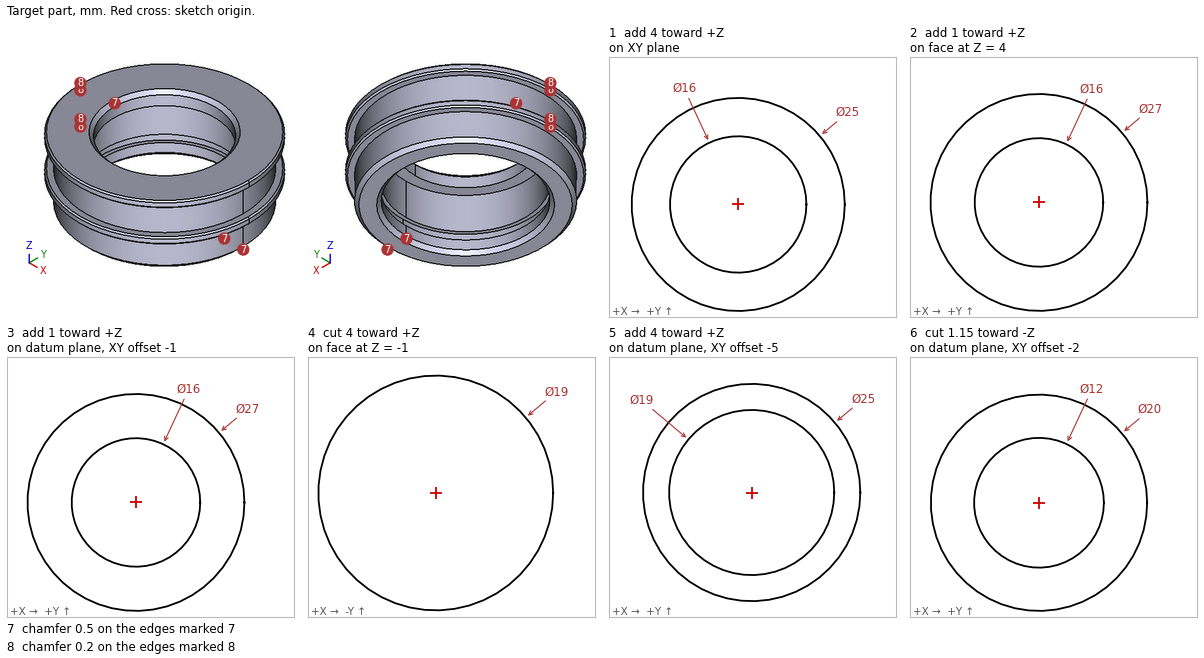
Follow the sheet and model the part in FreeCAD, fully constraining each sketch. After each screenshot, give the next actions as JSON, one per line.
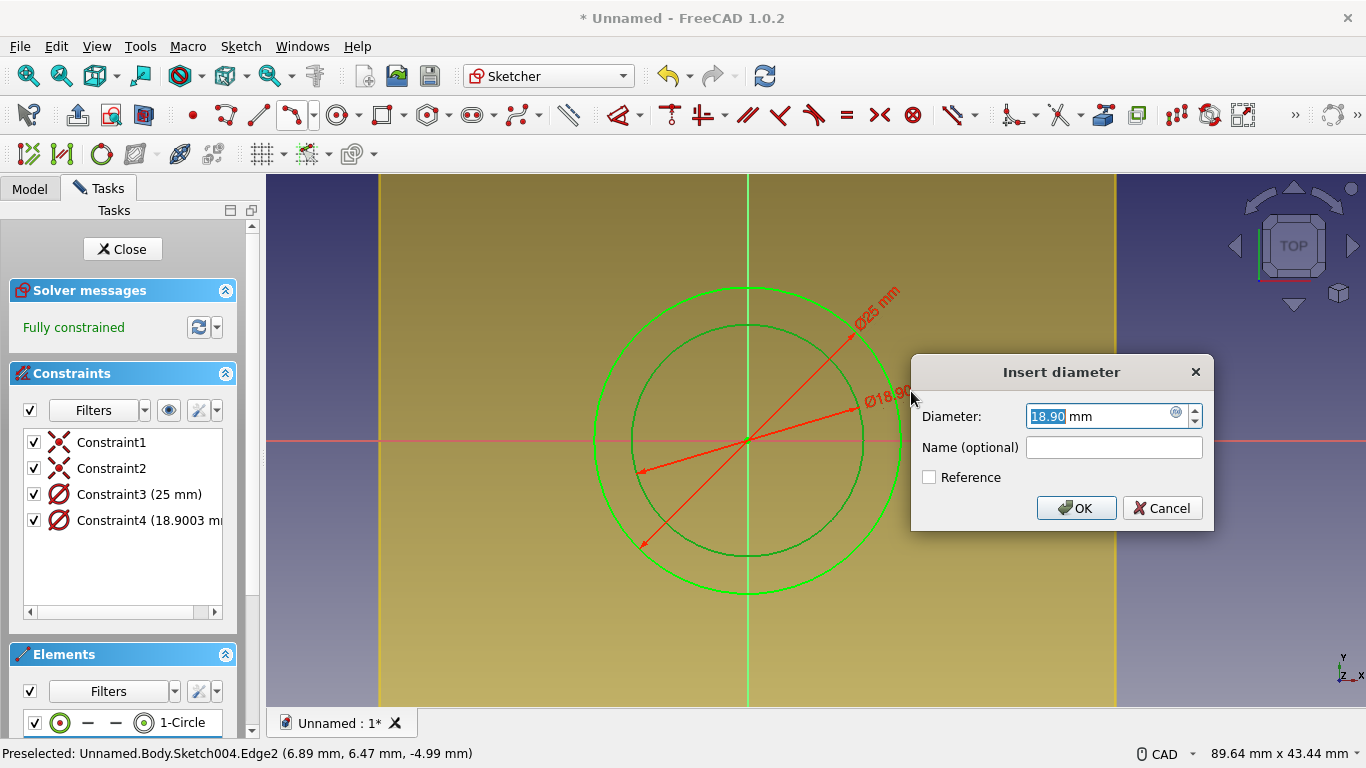
{"action": "type", "text": "19"}
{"action": "key", "text": "Return"}
{"action": "key", "text": "Escape"}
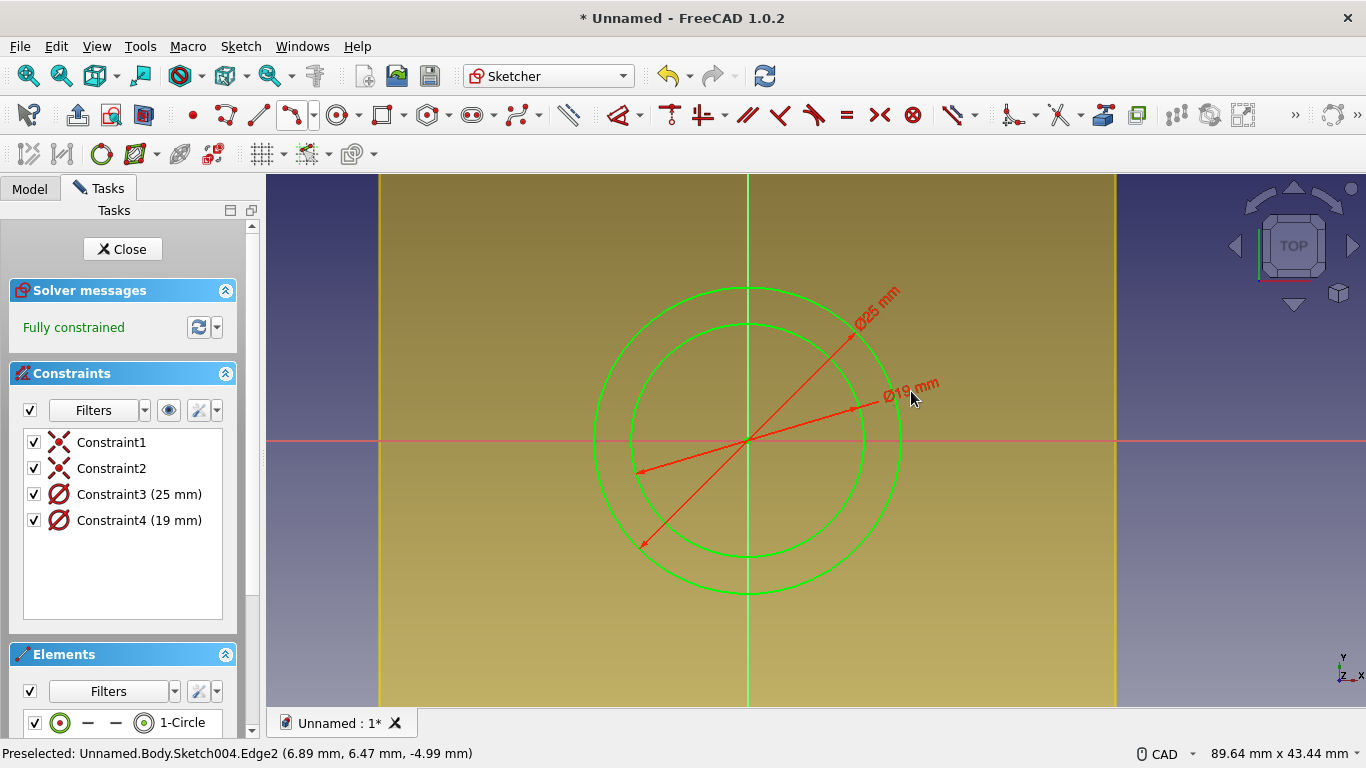
{"action": "left_click", "coordinate": [123, 249]}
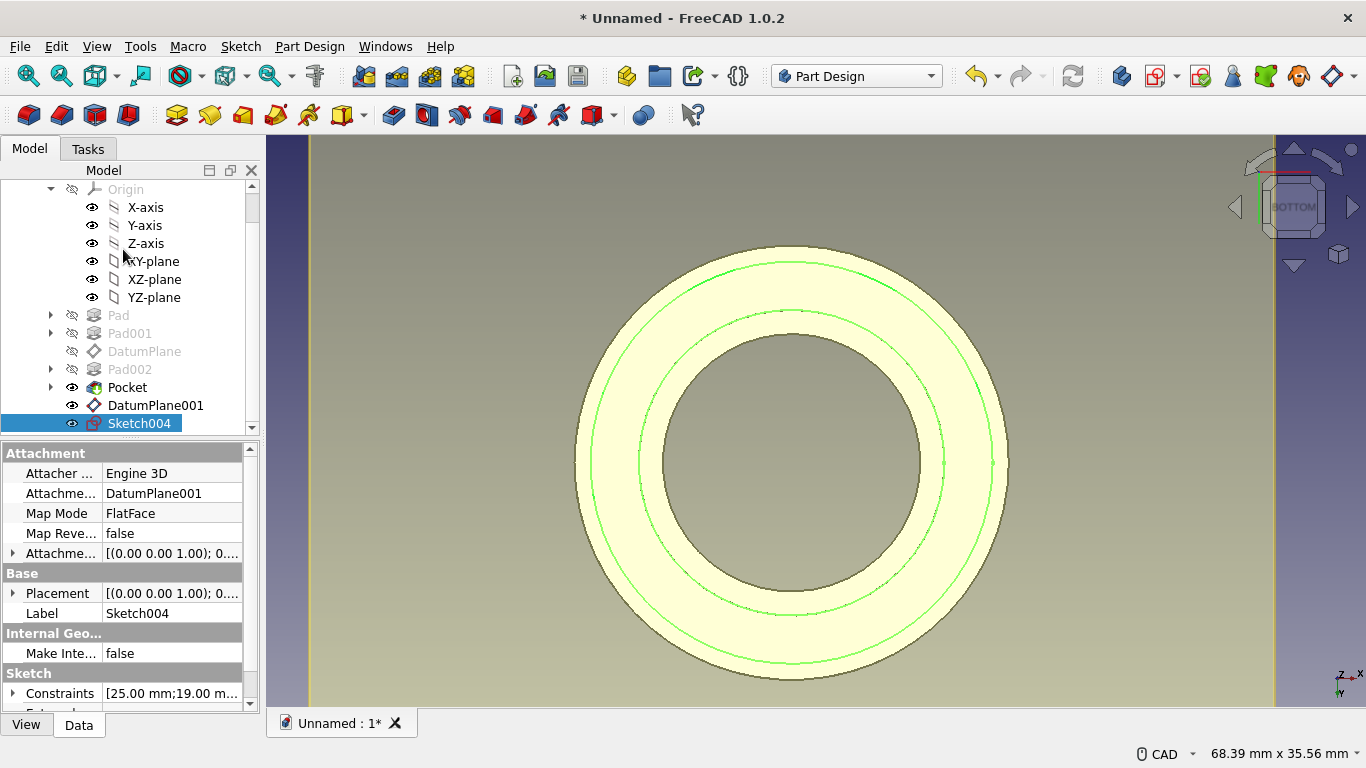
{"action": "left_click", "coordinate": [177, 116]}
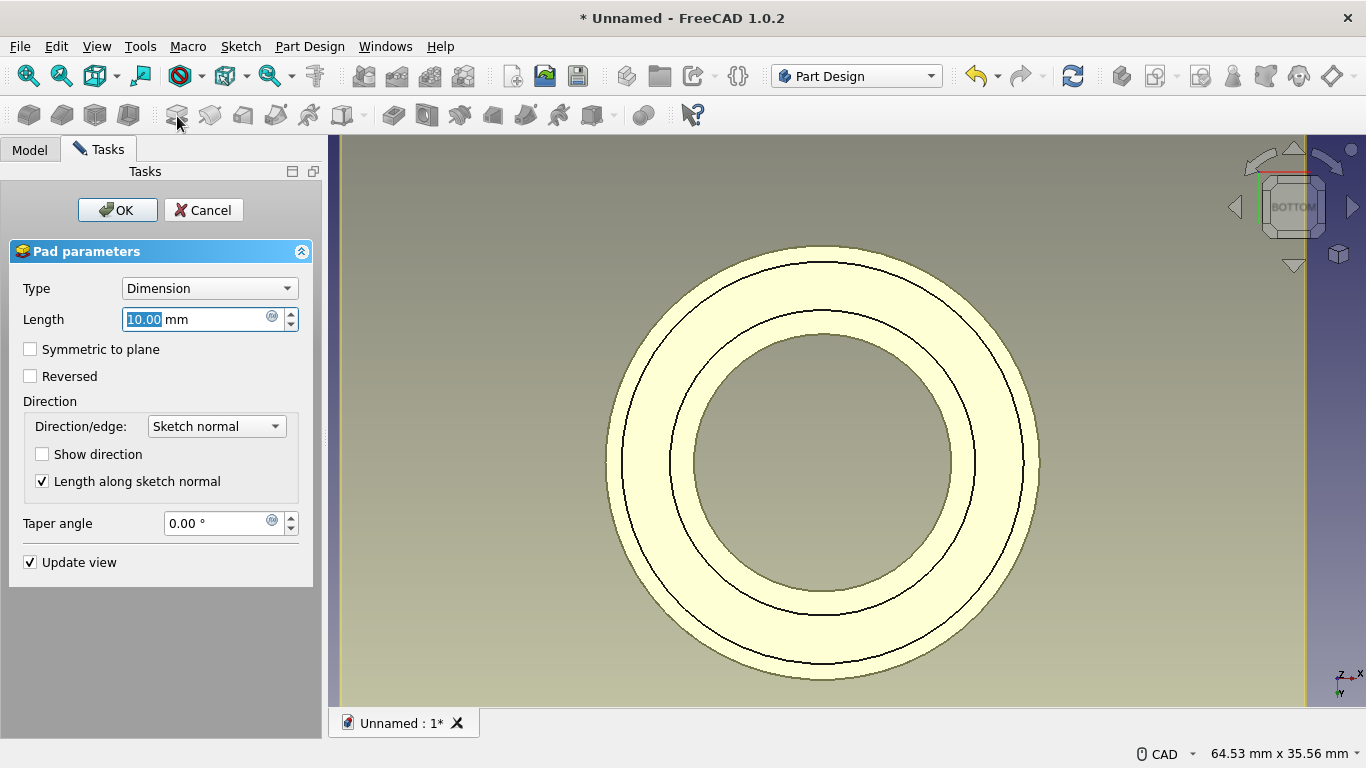
{"action": "type", "text": "4"}
{"action": "key", "text": "Tab"}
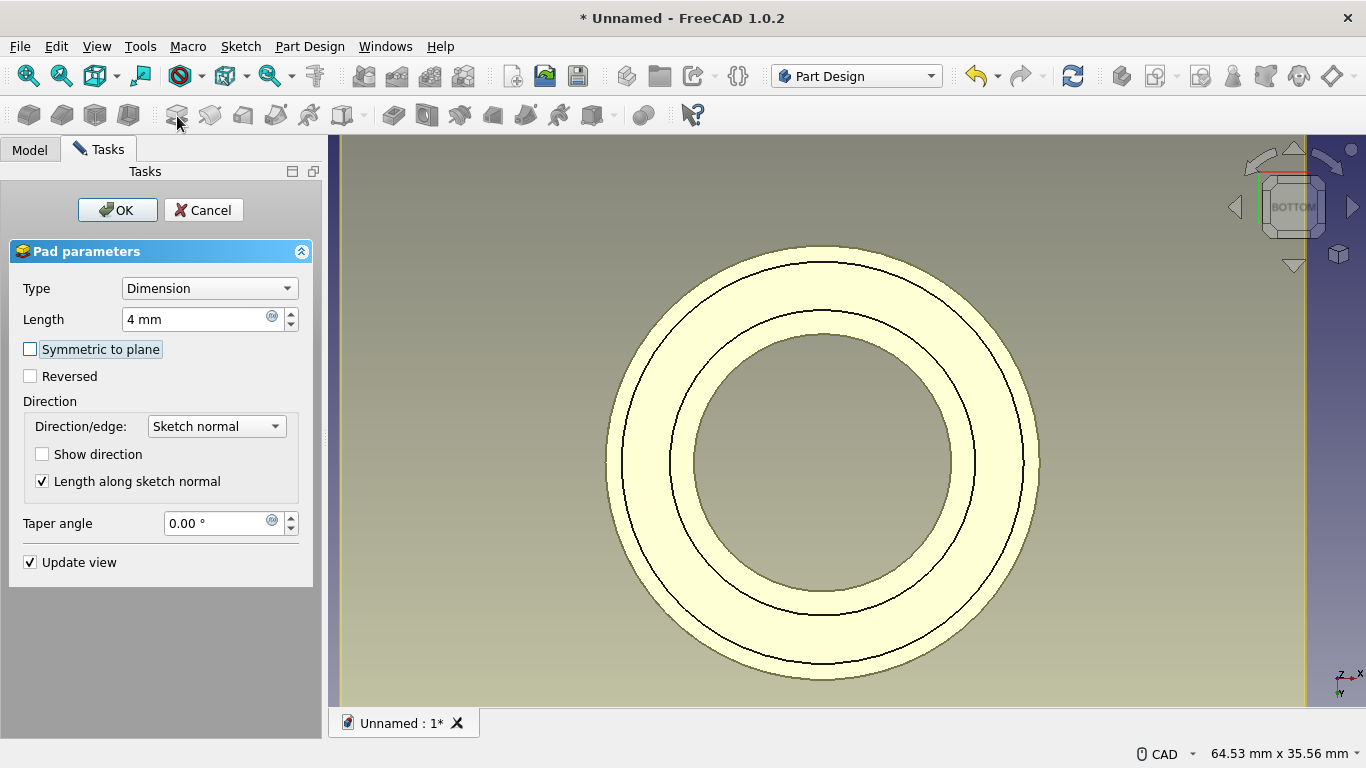
{"action": "left_click", "coordinate": [118, 210]}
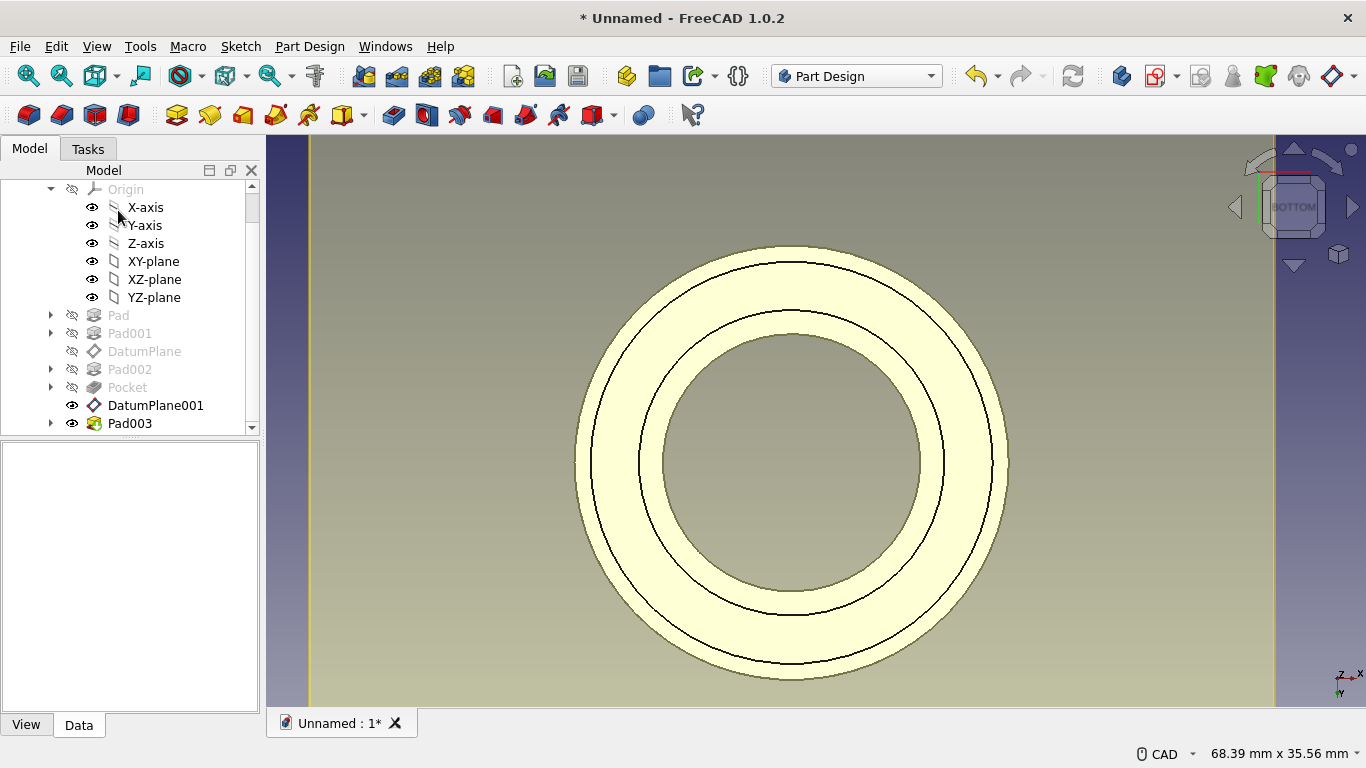
{"action": "left_click", "coordinate": [117, 405]}
{"action": "key", "text": "space"}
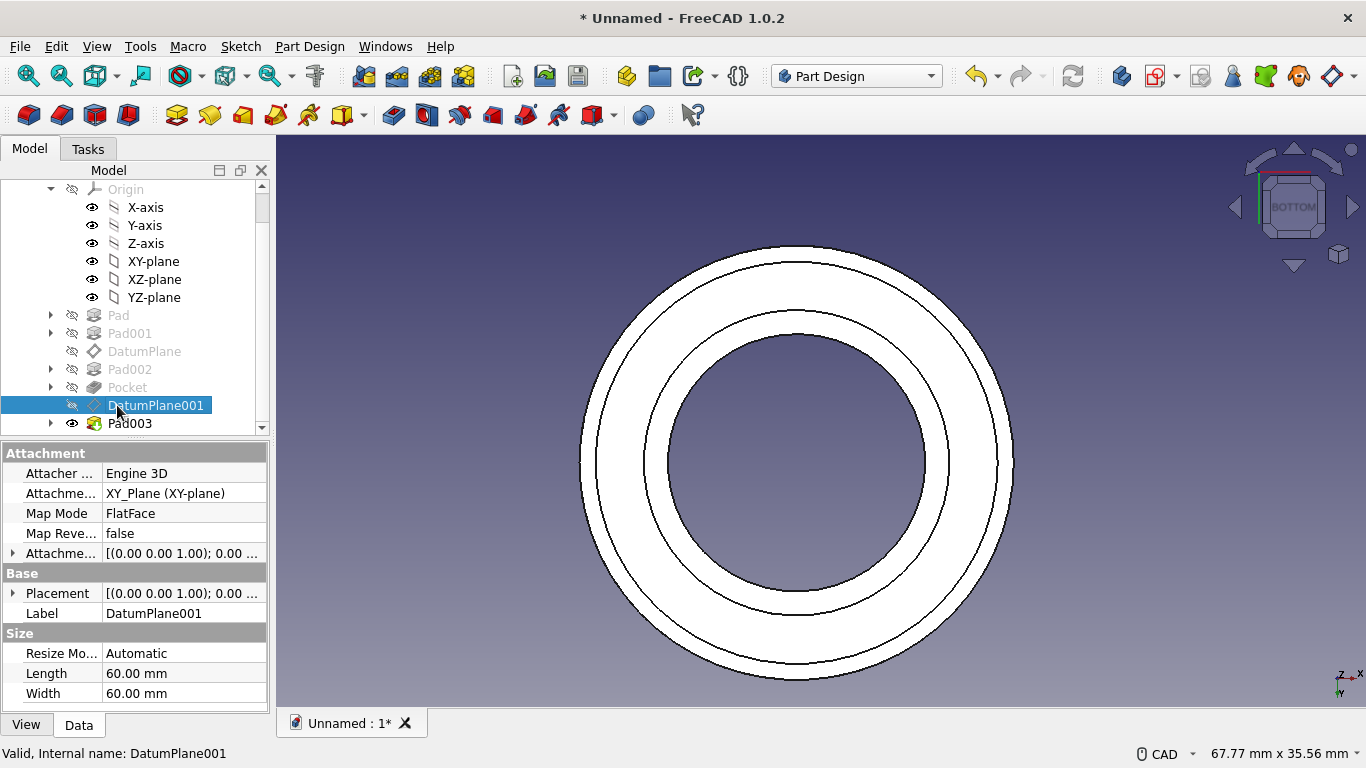
{"action": "left_click", "coordinate": [137, 261]}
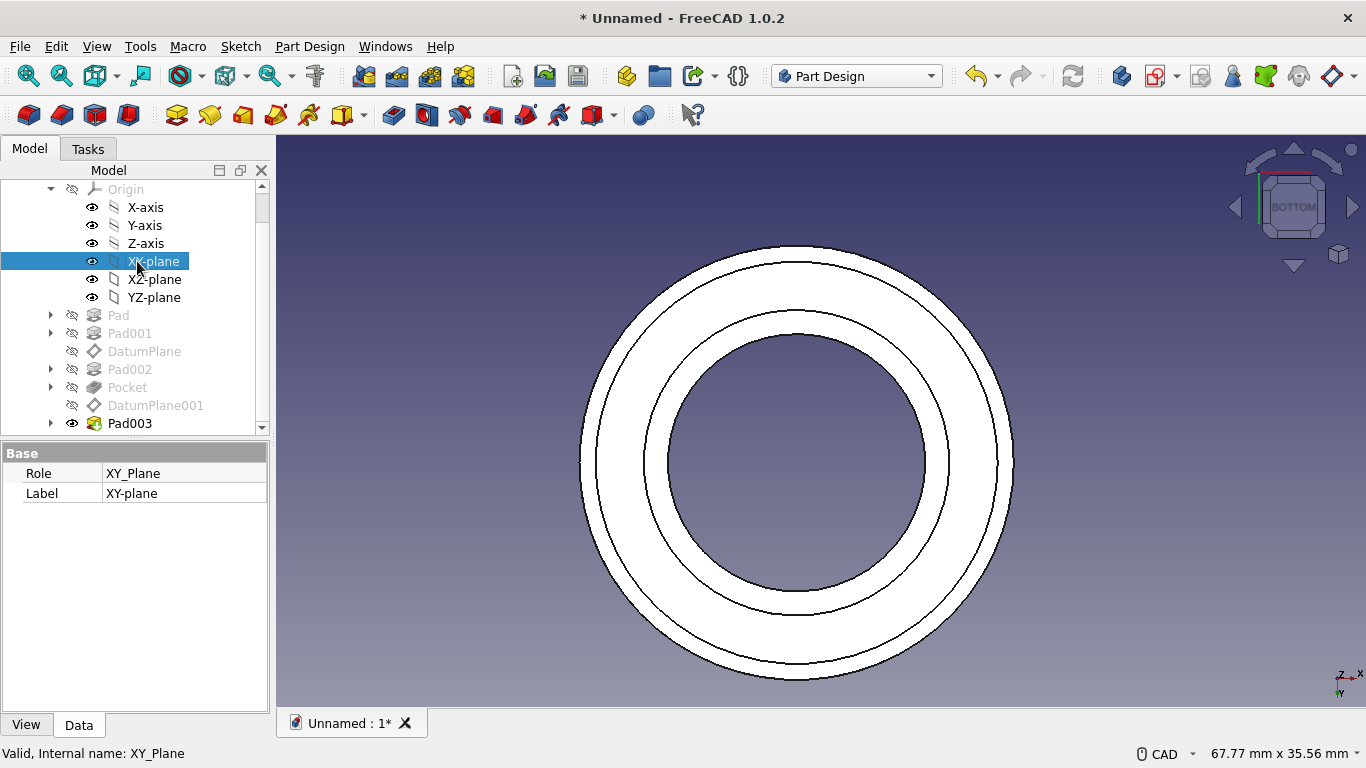
{"action": "left_click", "coordinate": [1332, 76]}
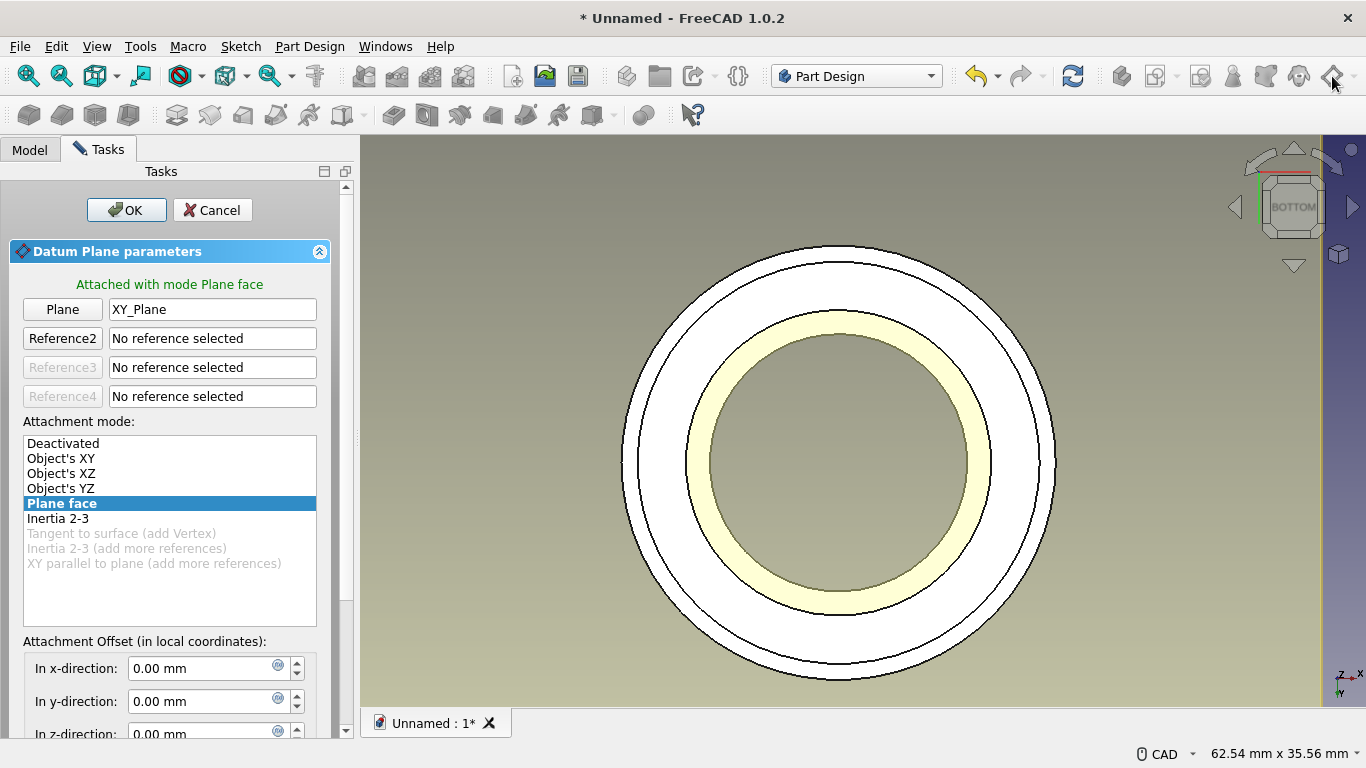
{"action": "scroll", "coordinate": [346, 460], "scroll_direction": "down", "scroll_amount": 2}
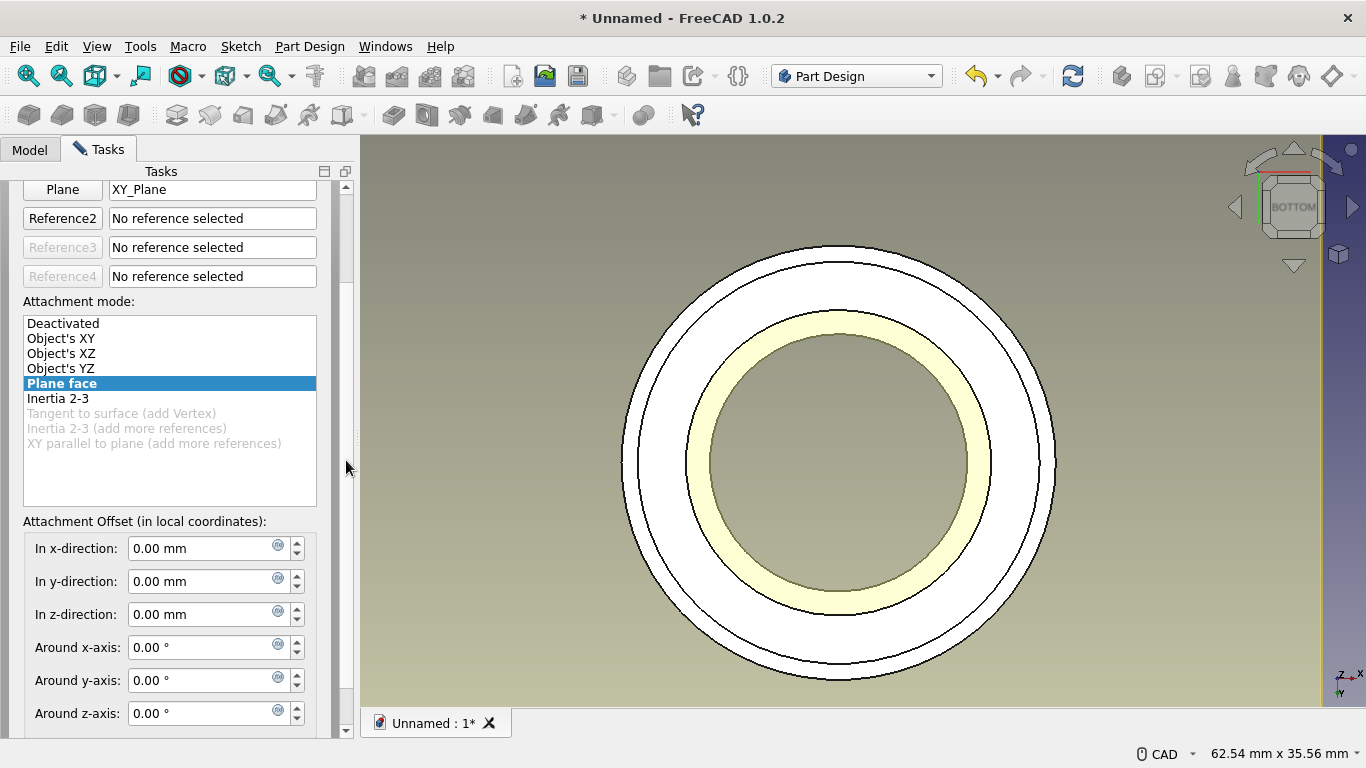
{"action": "triple_click", "coordinate": [210, 614]}